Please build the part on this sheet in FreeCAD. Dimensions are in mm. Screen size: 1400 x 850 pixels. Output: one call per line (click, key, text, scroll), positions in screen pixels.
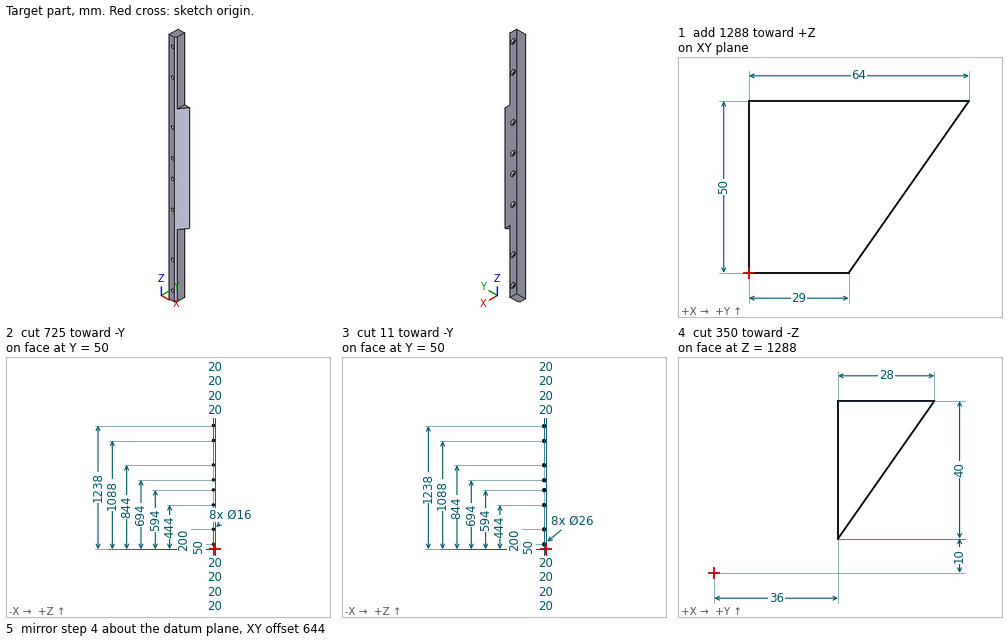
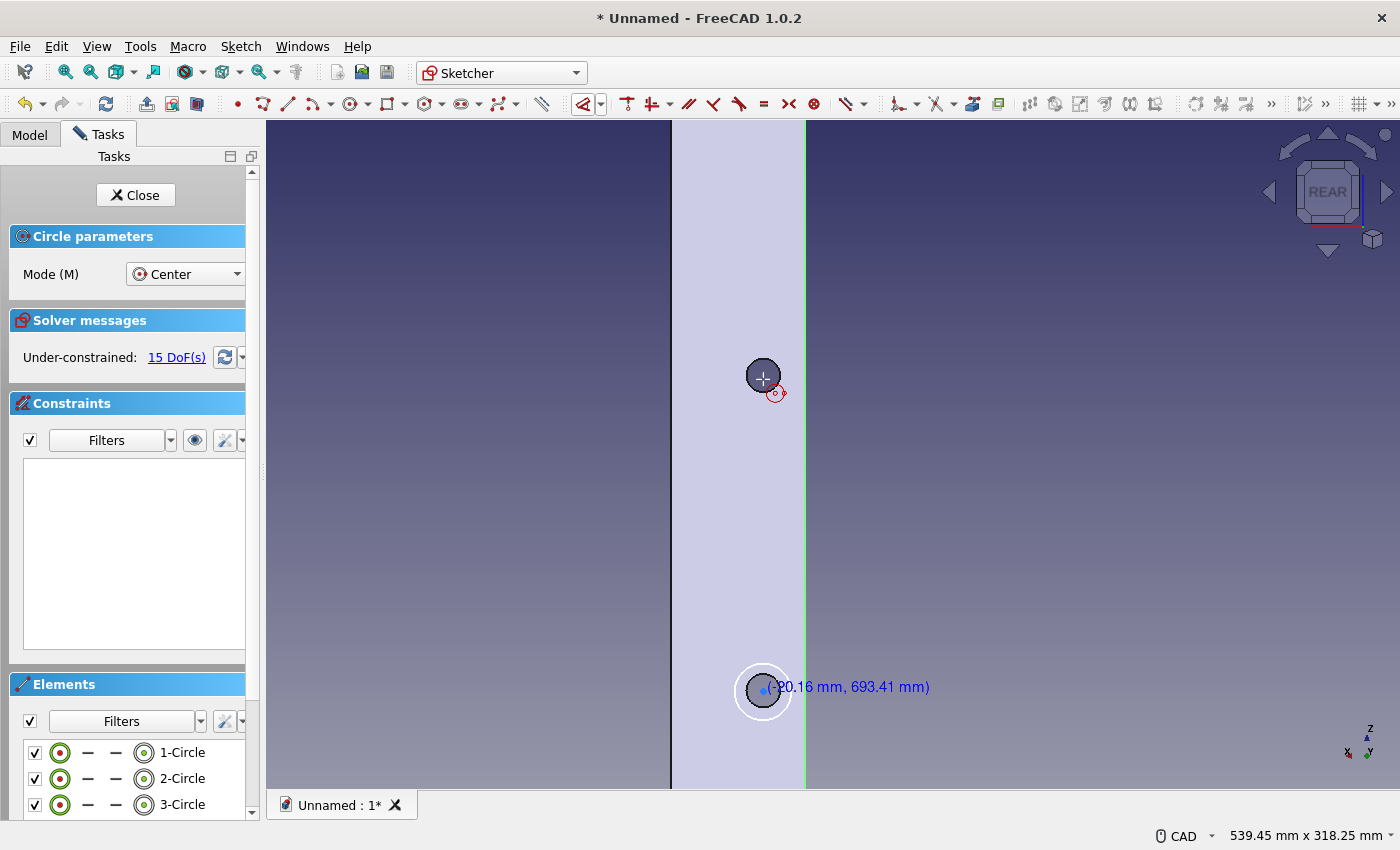
click(763, 375)
click(783, 356)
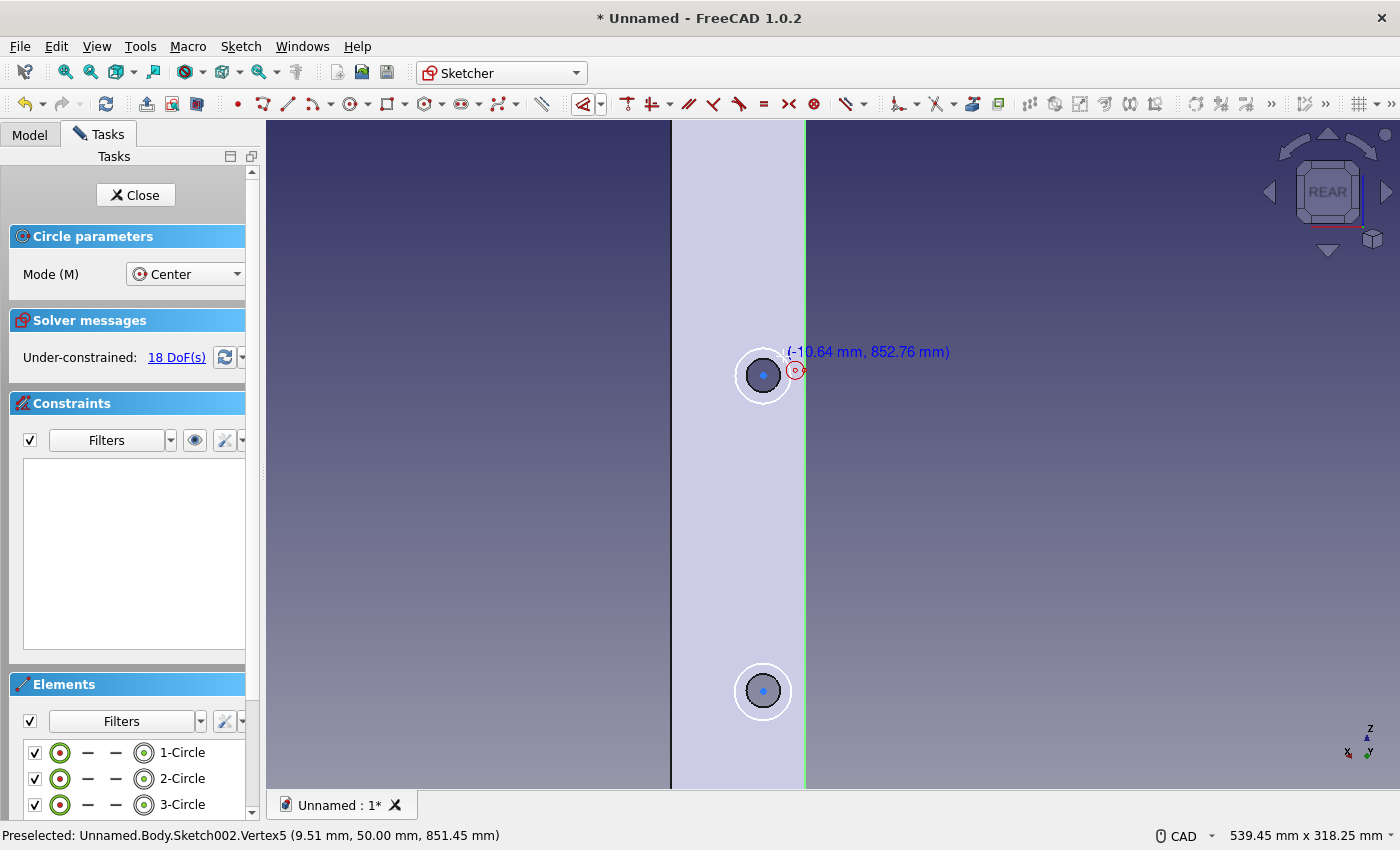
scroll(763, 379, down, 9)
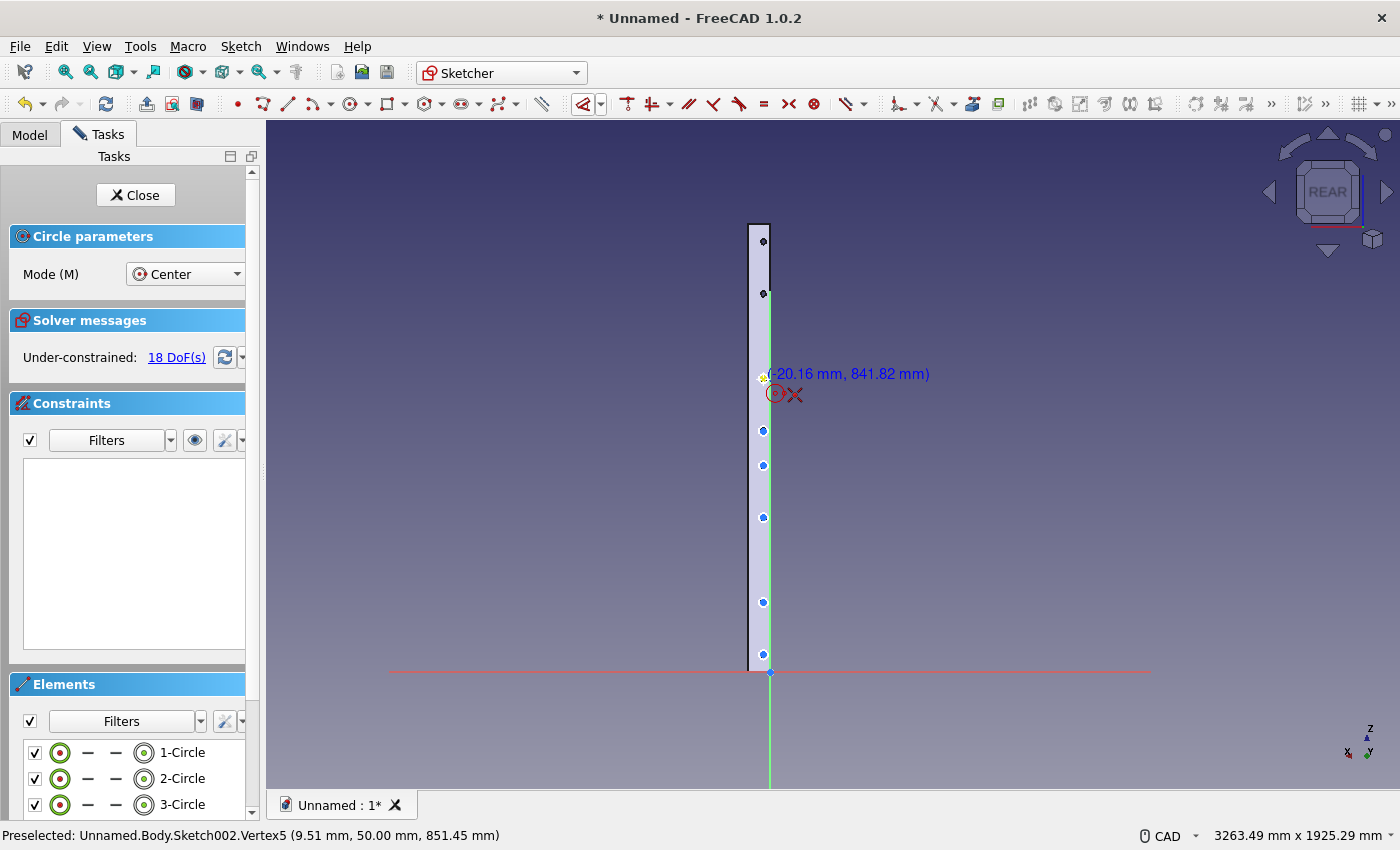
scroll(763, 294, up, 9)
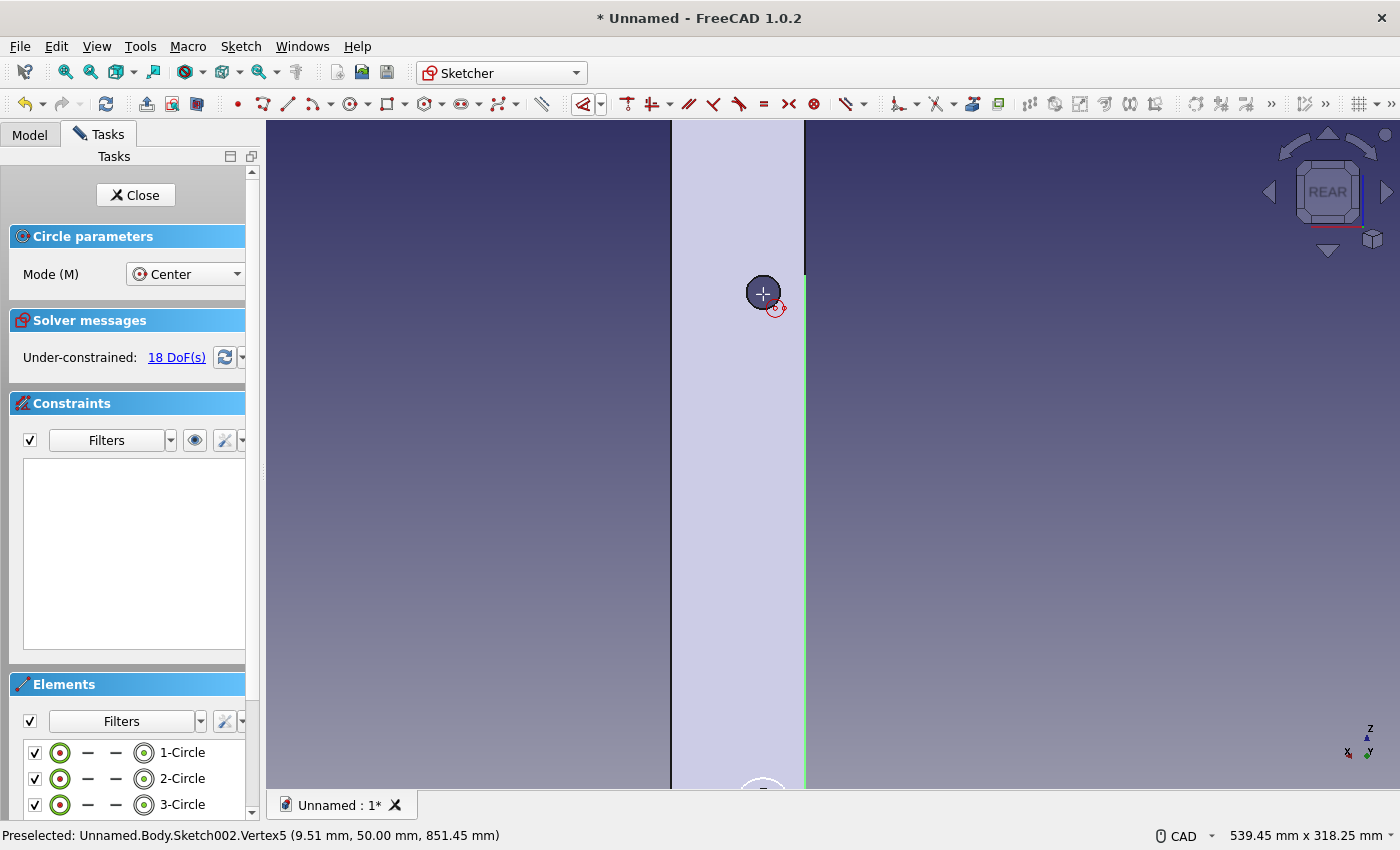
click(763, 292)
click(783, 273)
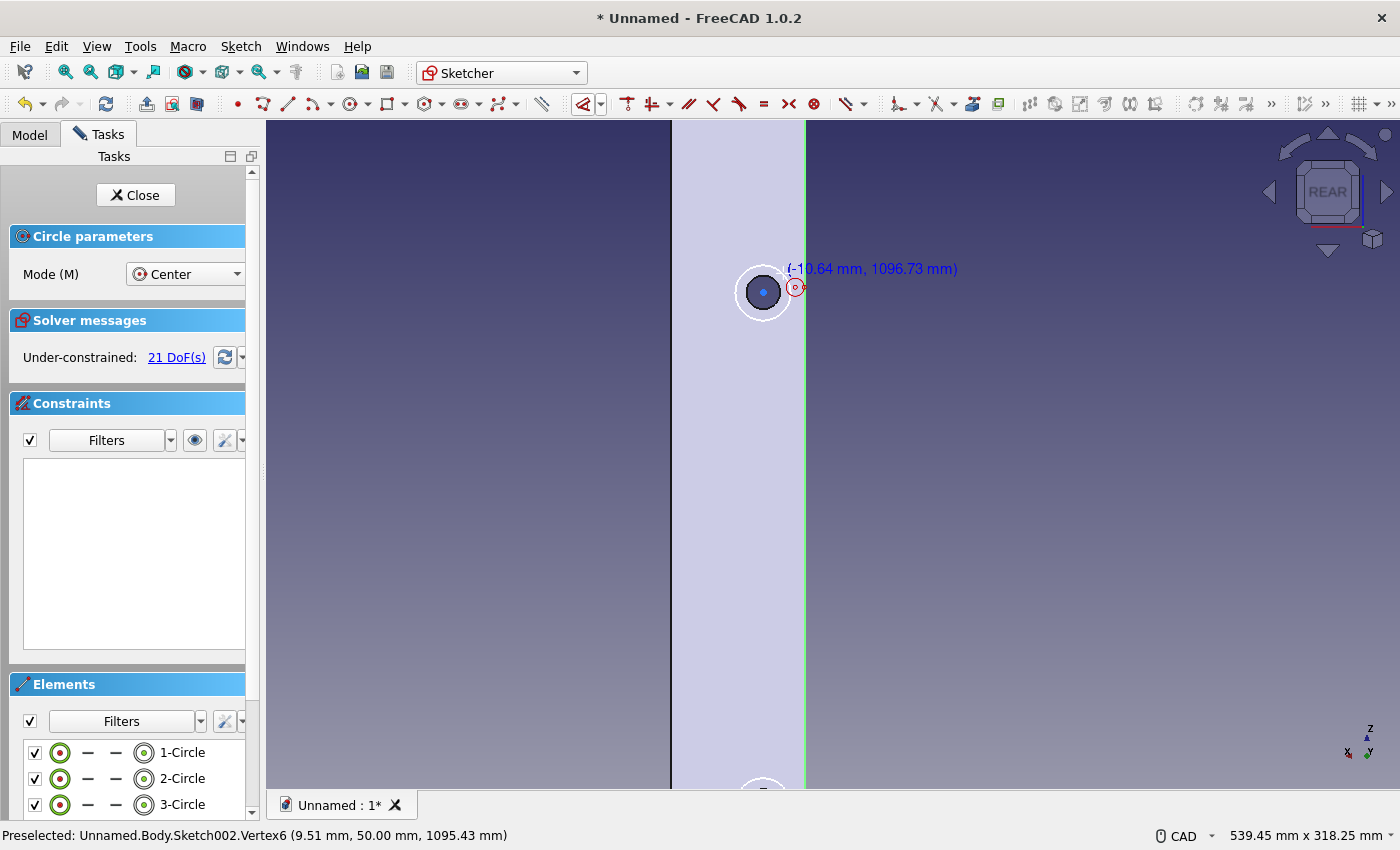
scroll(763, 294, down, 9)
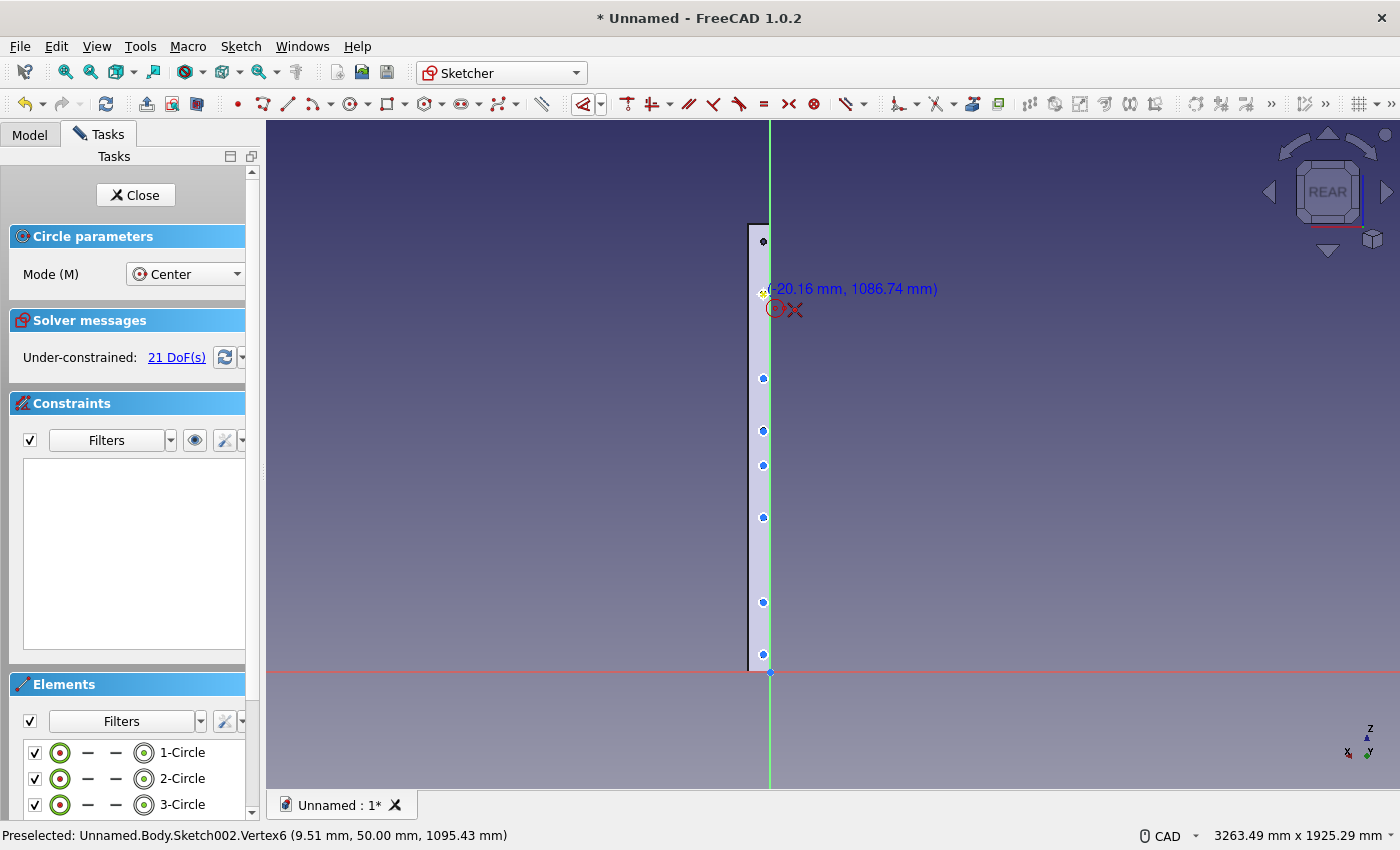
scroll(763, 242, up, 9)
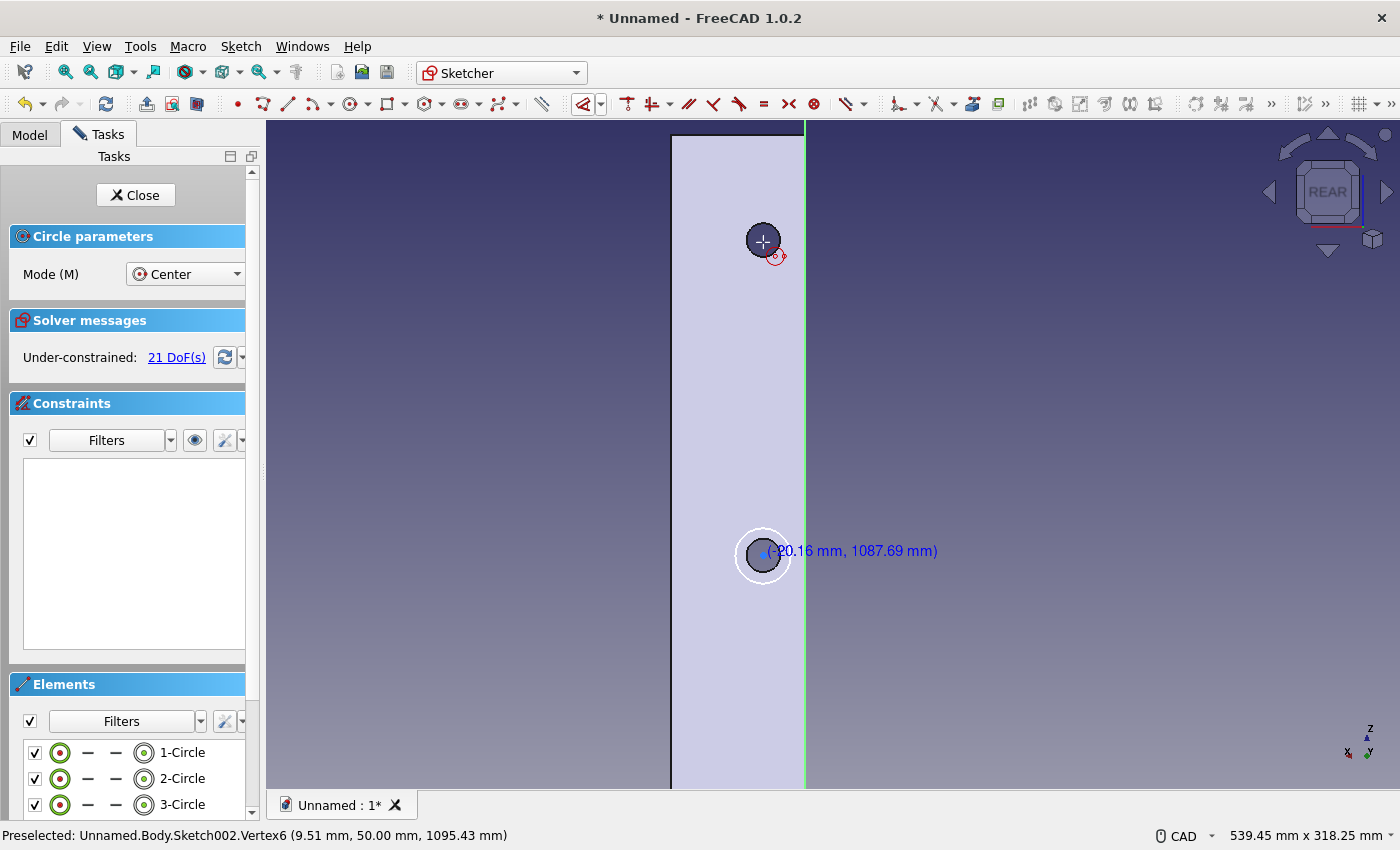
click(763, 240)
click(783, 221)
key(Escape)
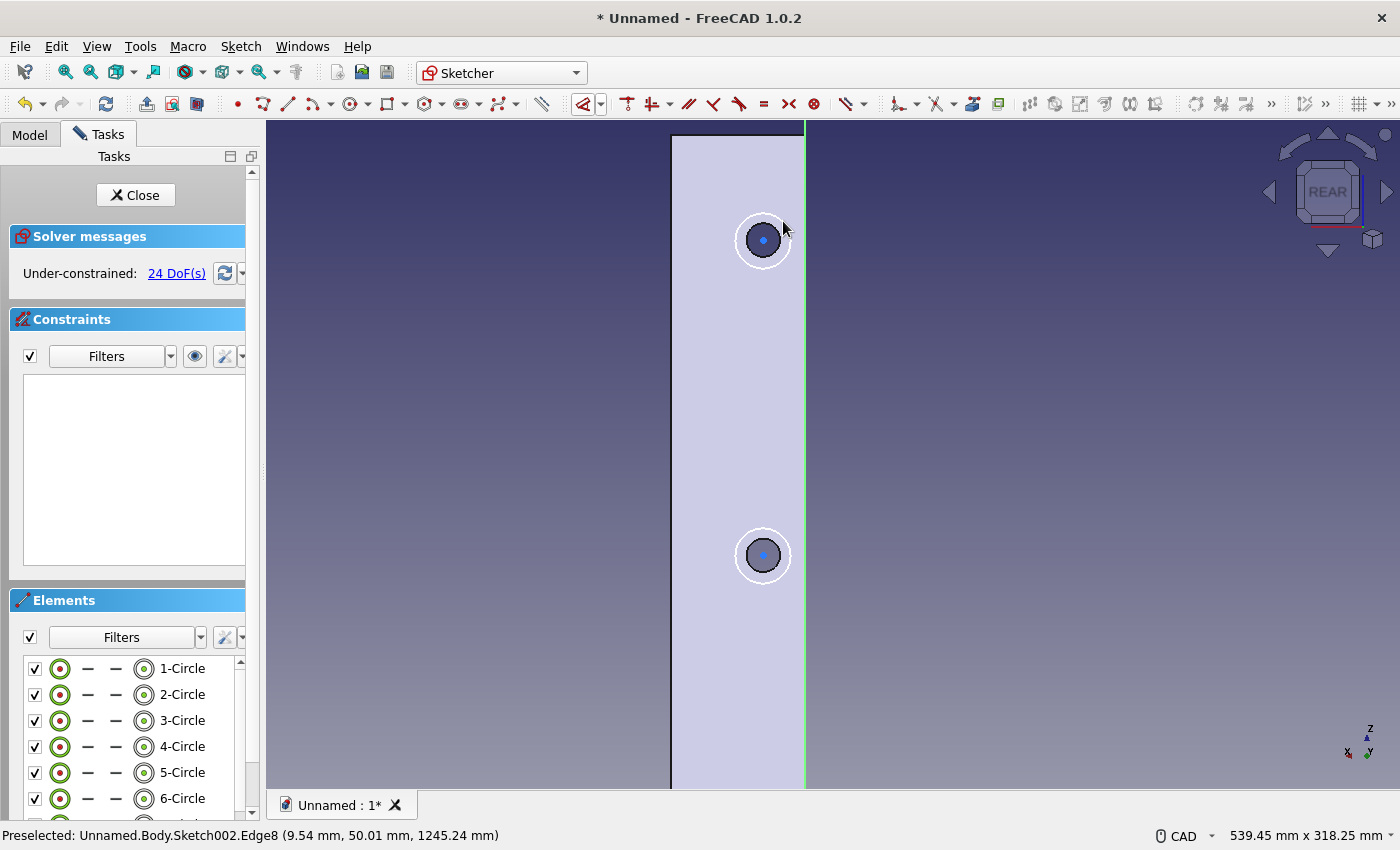
scroll(763, 242, down, 9)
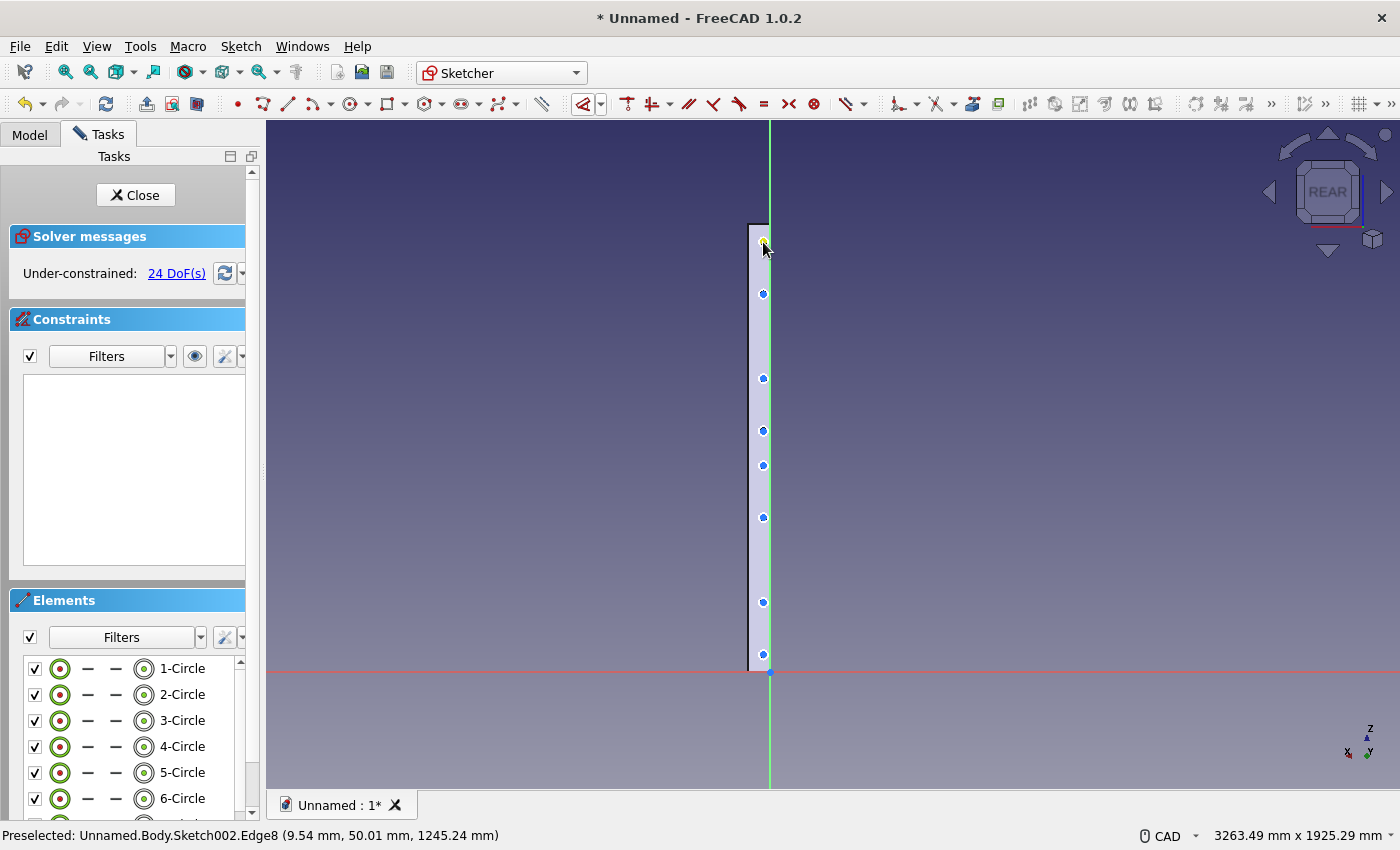
scroll(767, 652, up, 7)